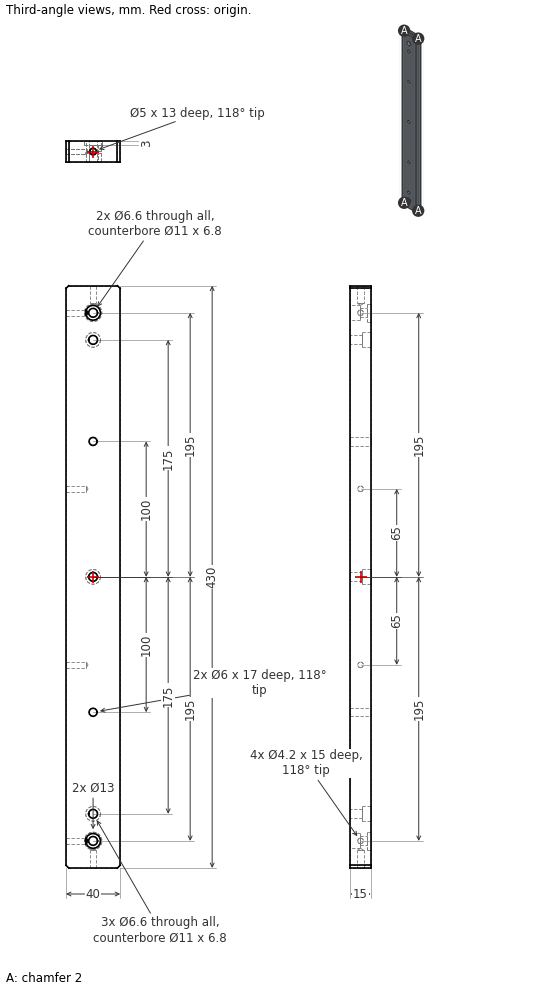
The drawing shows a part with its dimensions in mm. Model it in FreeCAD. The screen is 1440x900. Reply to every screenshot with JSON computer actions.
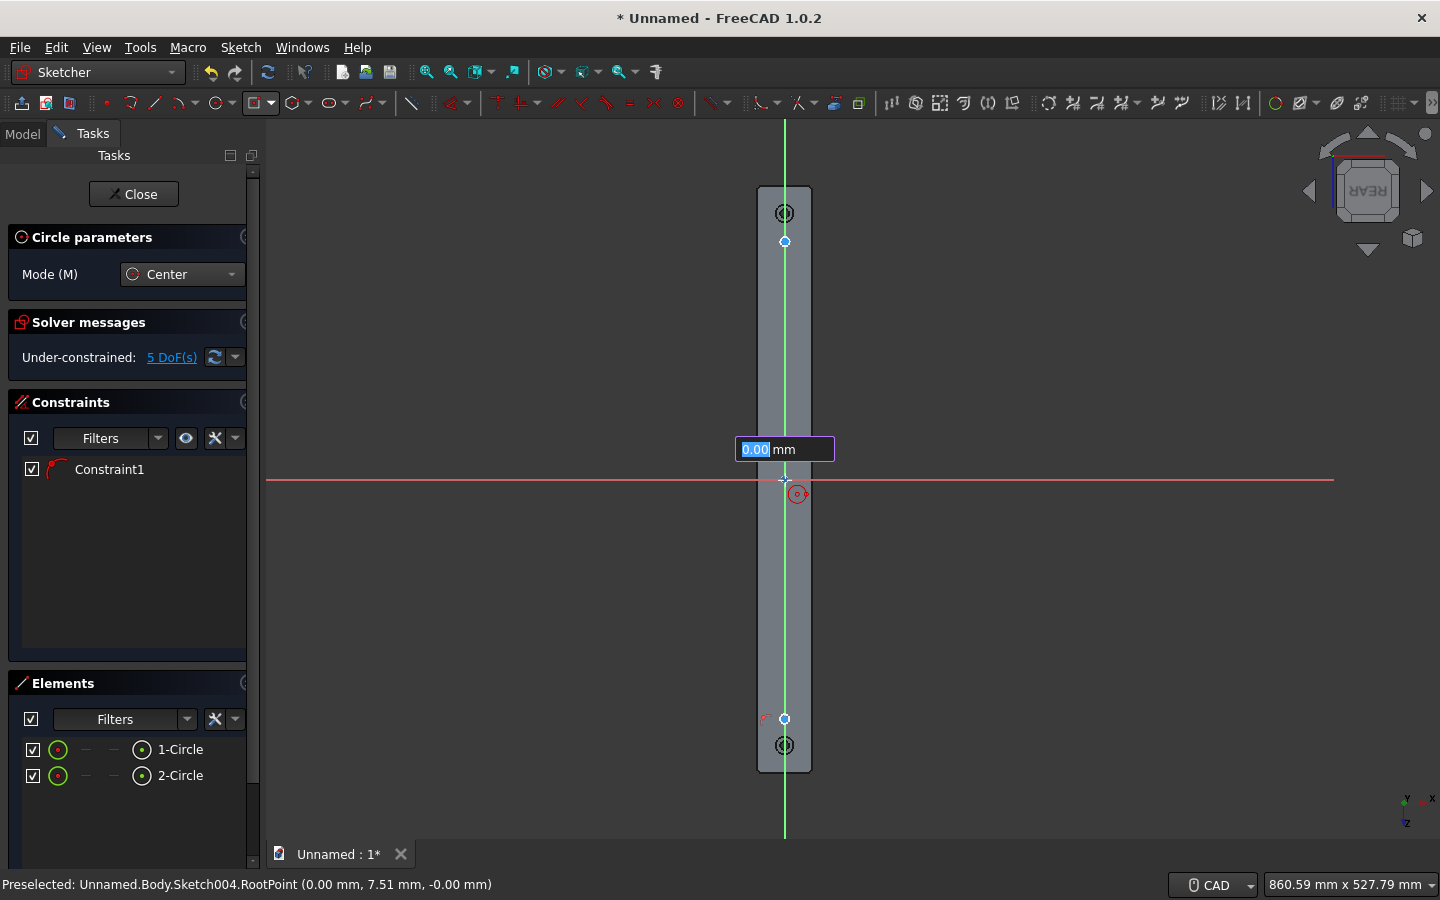
{"action": "scroll", "coordinate": [788, 476], "scroll_direction": "up", "scroll_amount": 9}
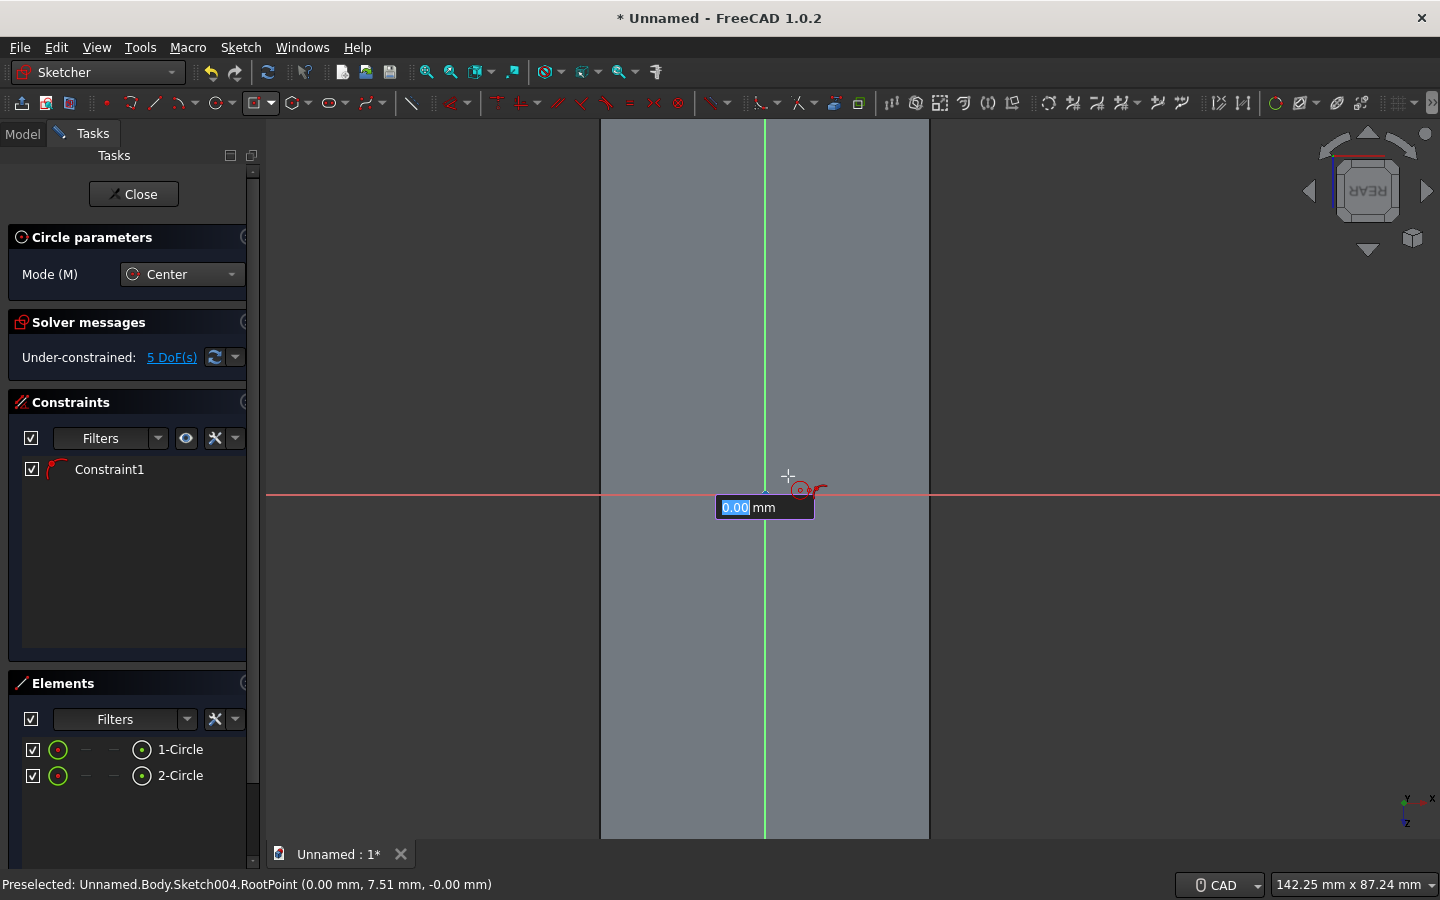
{"action": "left_click", "coordinate": [784, 475]}
{"action": "key", "text": "Escape"}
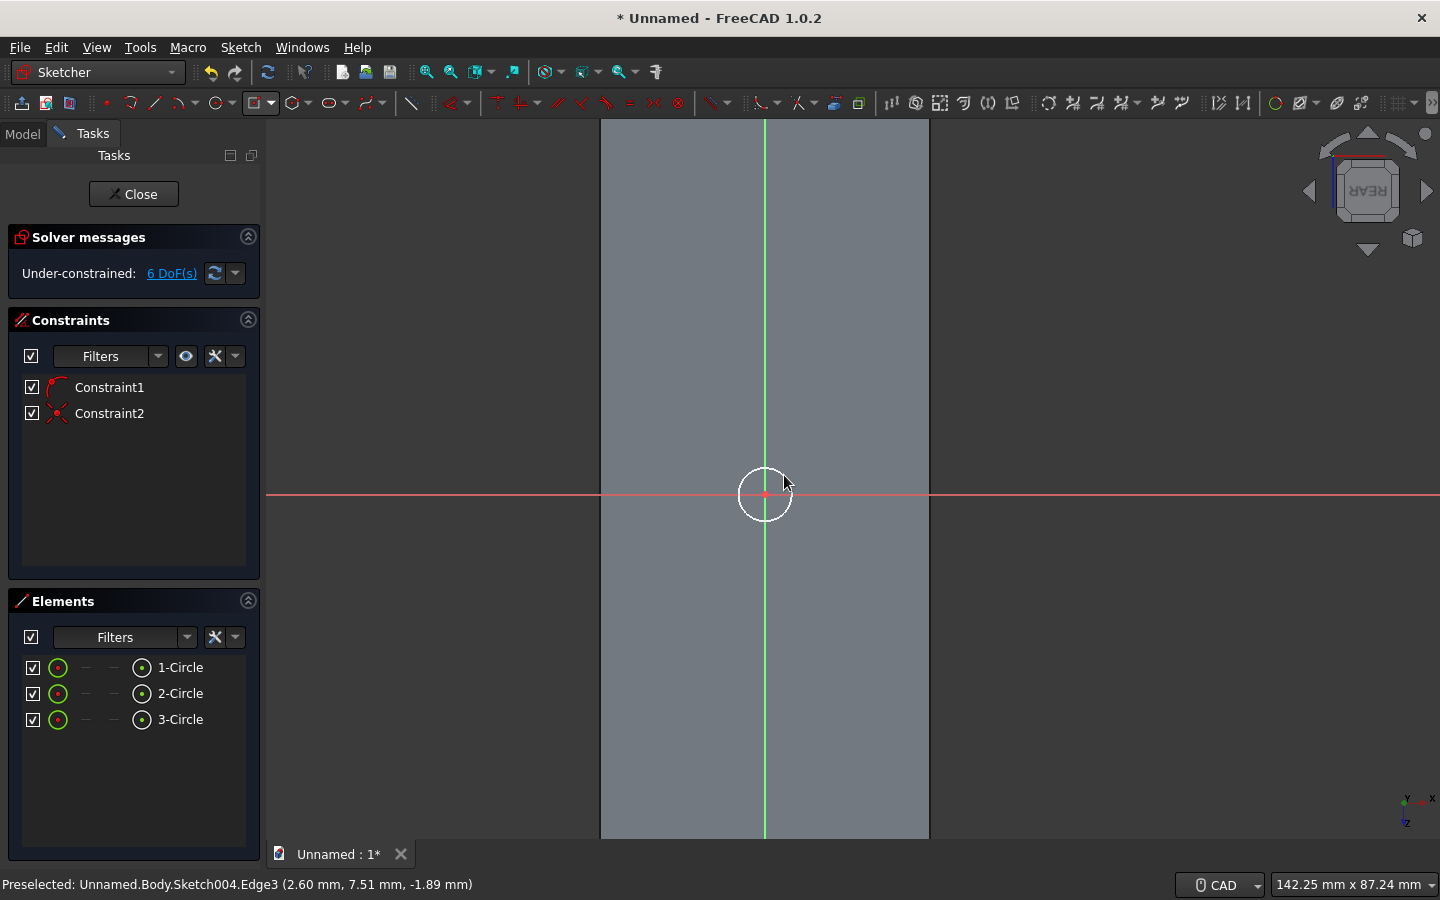
{"action": "scroll", "coordinate": [788, 476], "scroll_direction": "down", "scroll_amount": 9}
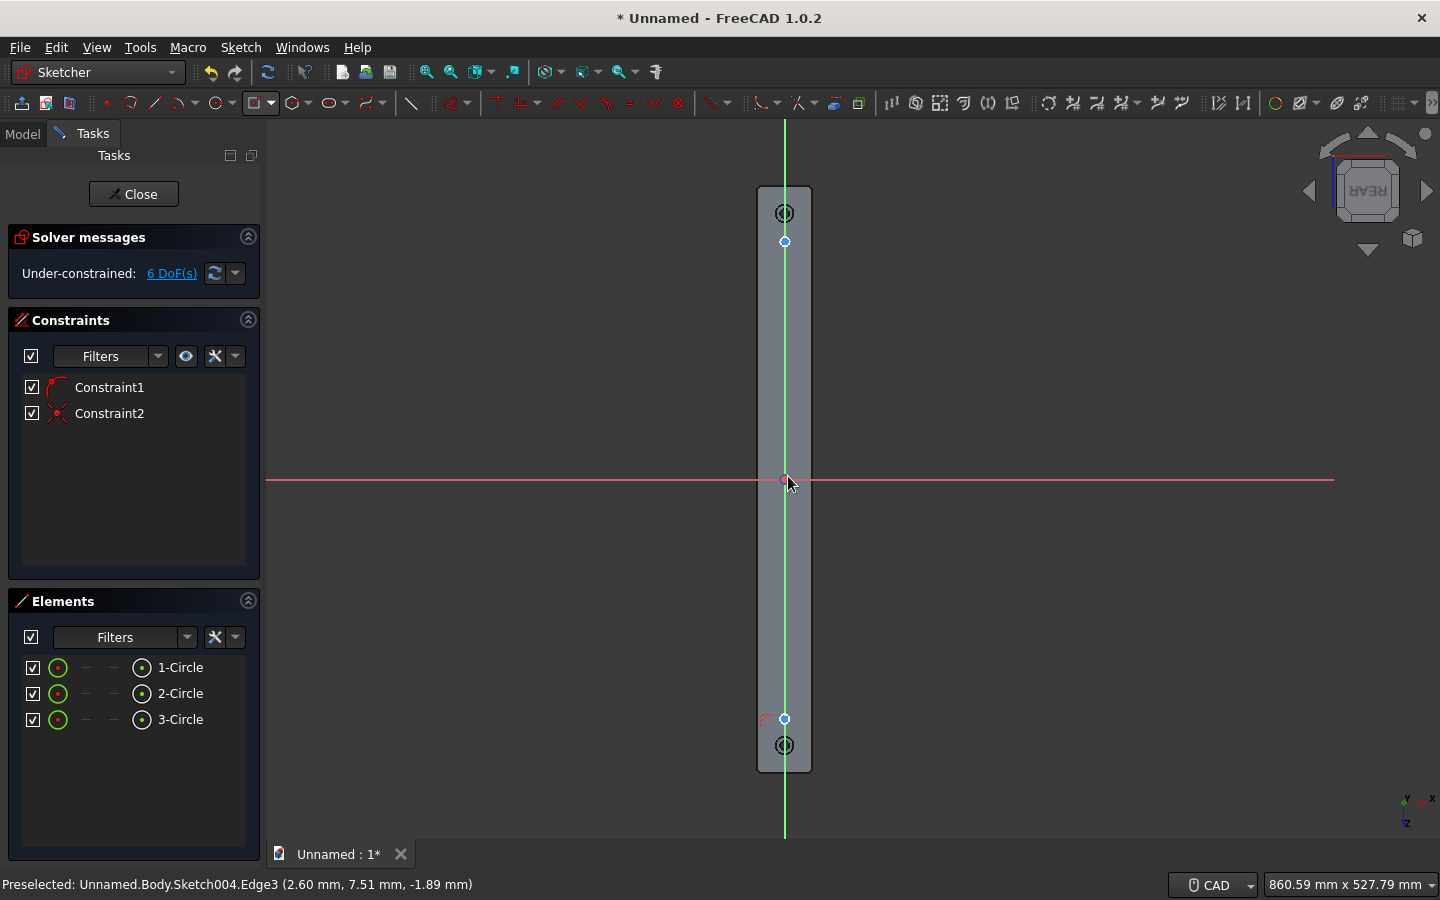
{"action": "scroll", "coordinate": [788, 239], "scroll_direction": "up", "scroll_amount": 7}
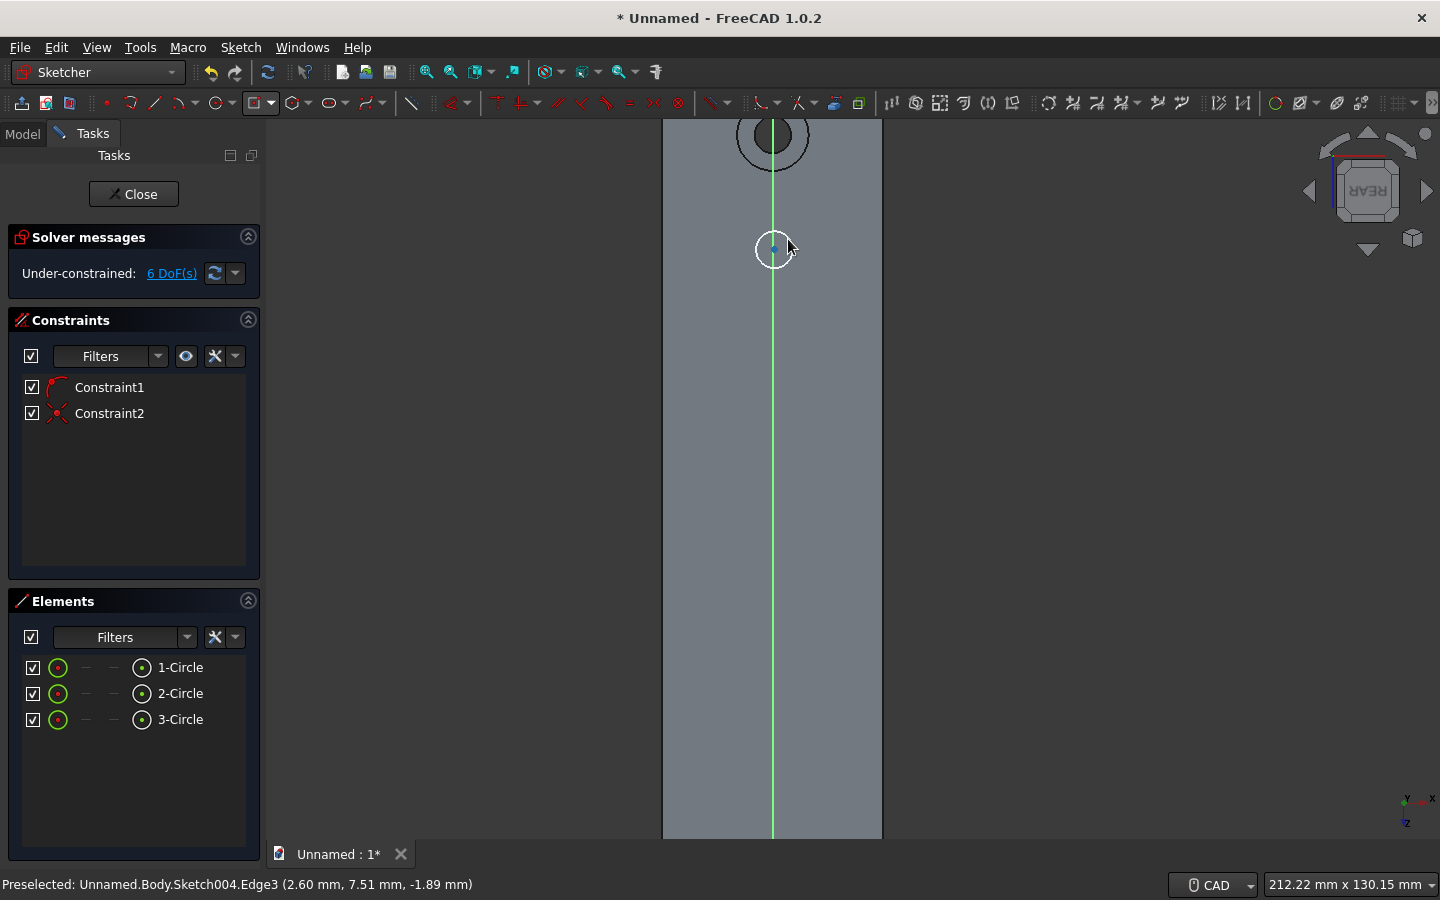
{"action": "left_click", "coordinate": [787, 237]}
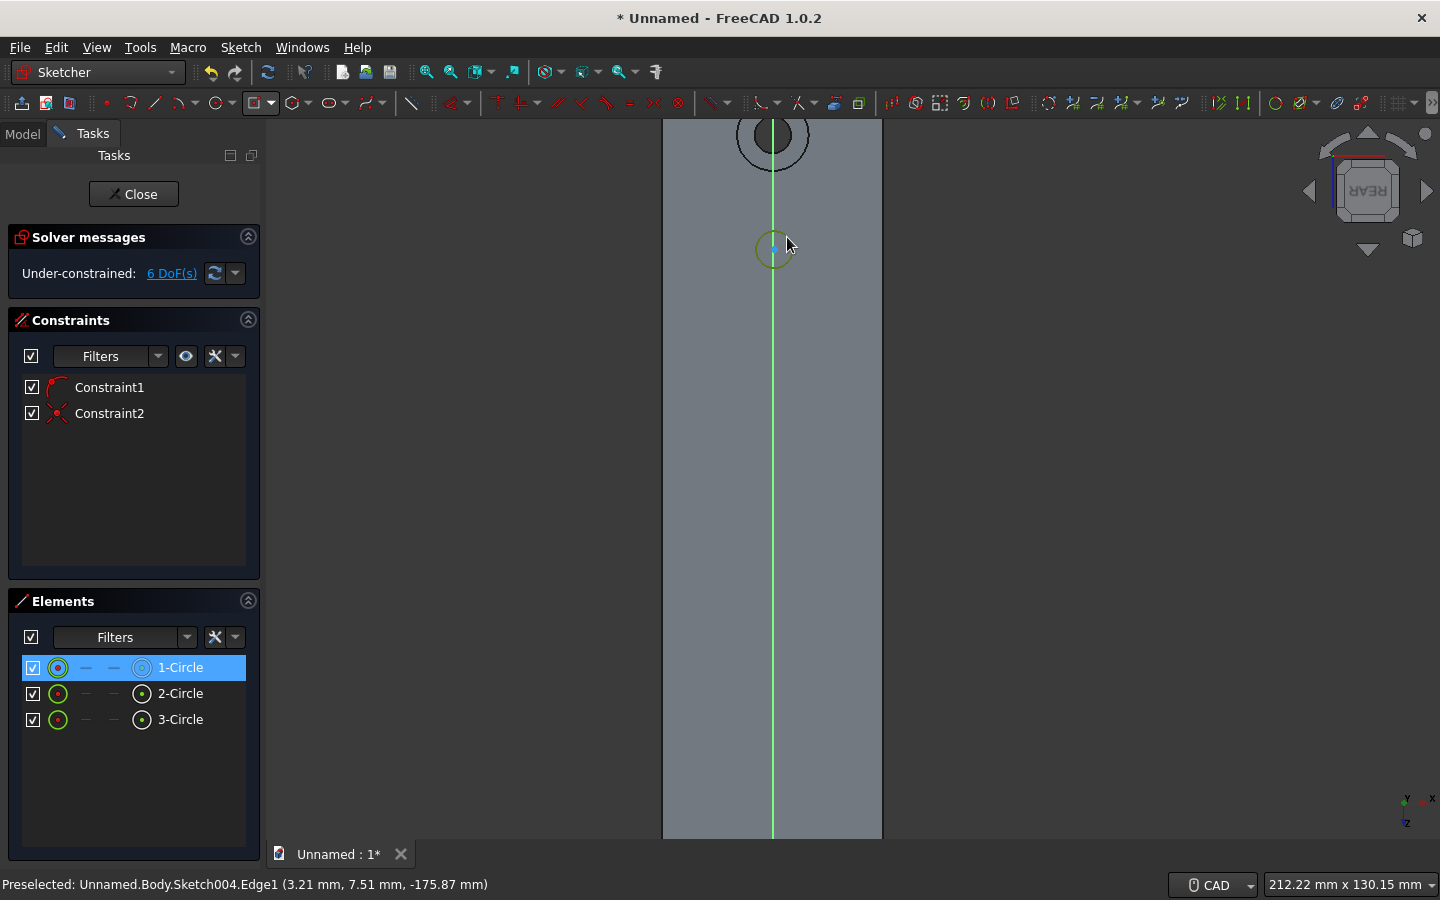
{"action": "scroll", "coordinate": [788, 239], "scroll_direction": "down", "scroll_amount": 7}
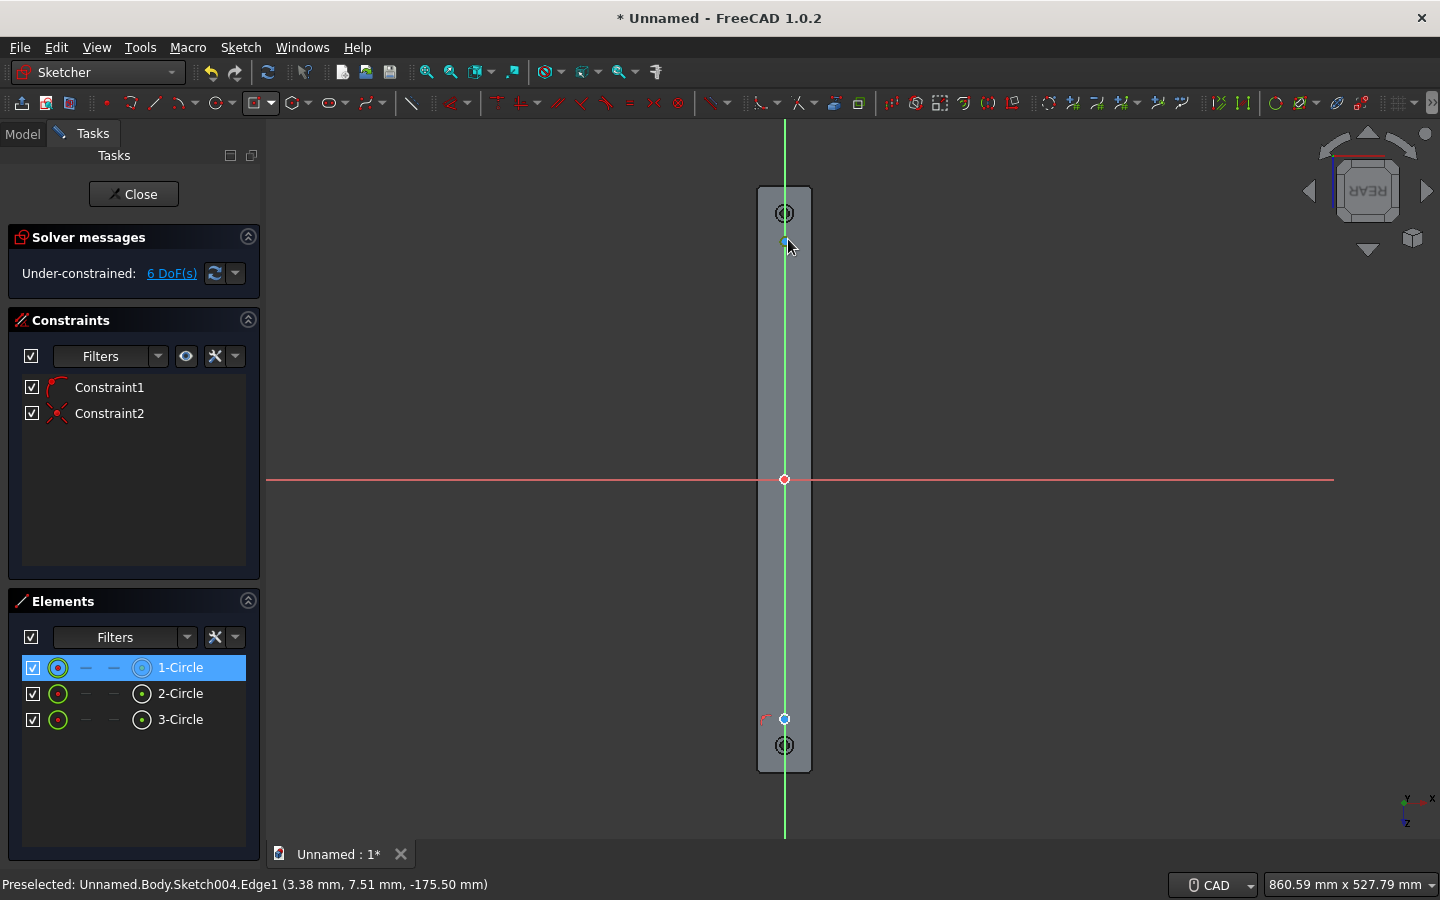
{"action": "scroll", "coordinate": [788, 716], "scroll_direction": "up", "scroll_amount": 8}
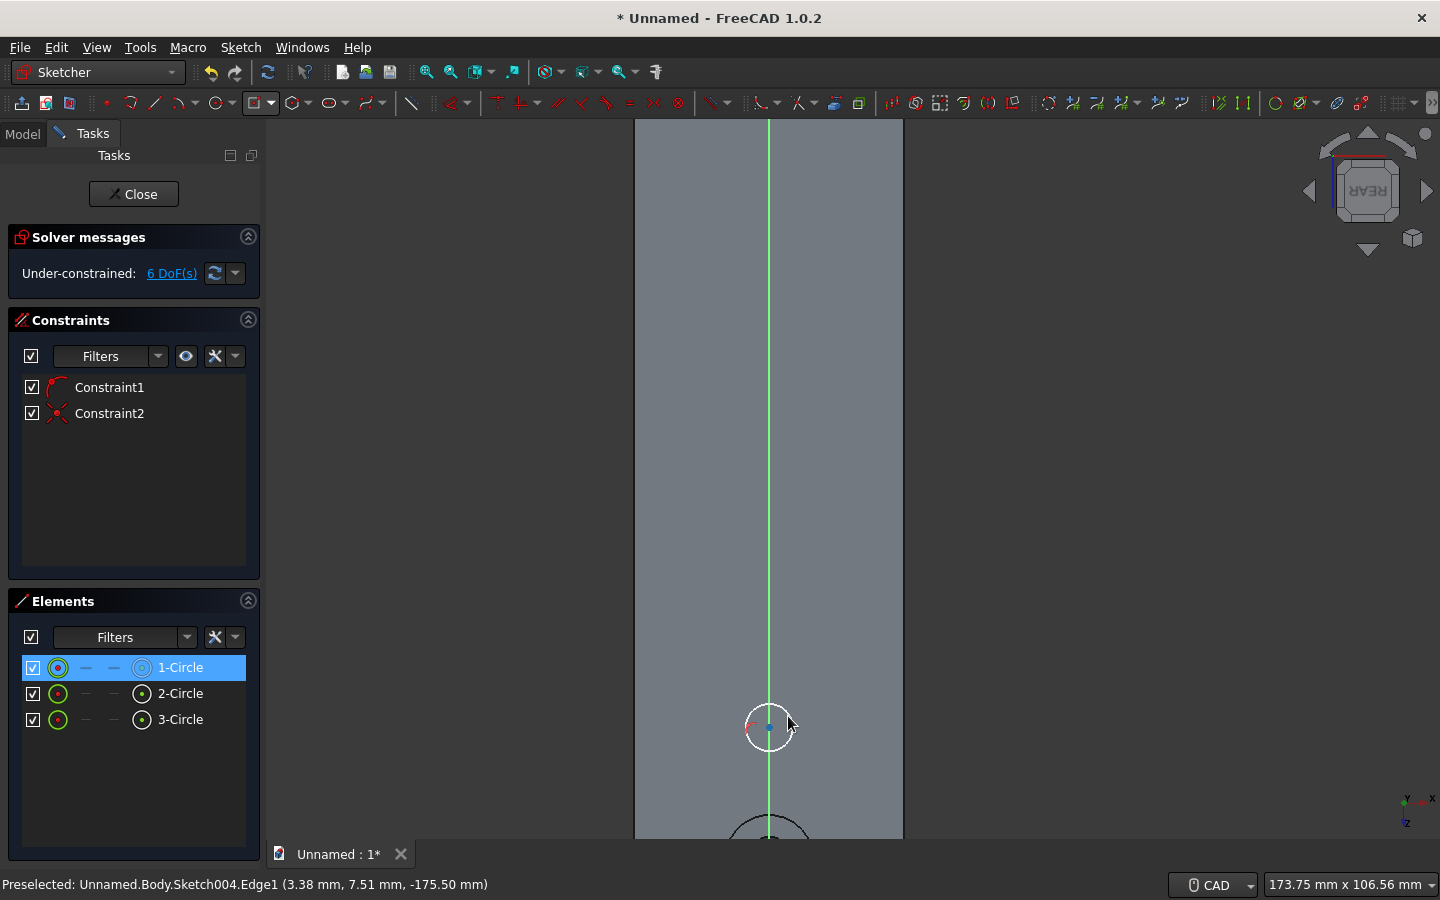
{"action": "left_click", "coordinate": [786, 711]}